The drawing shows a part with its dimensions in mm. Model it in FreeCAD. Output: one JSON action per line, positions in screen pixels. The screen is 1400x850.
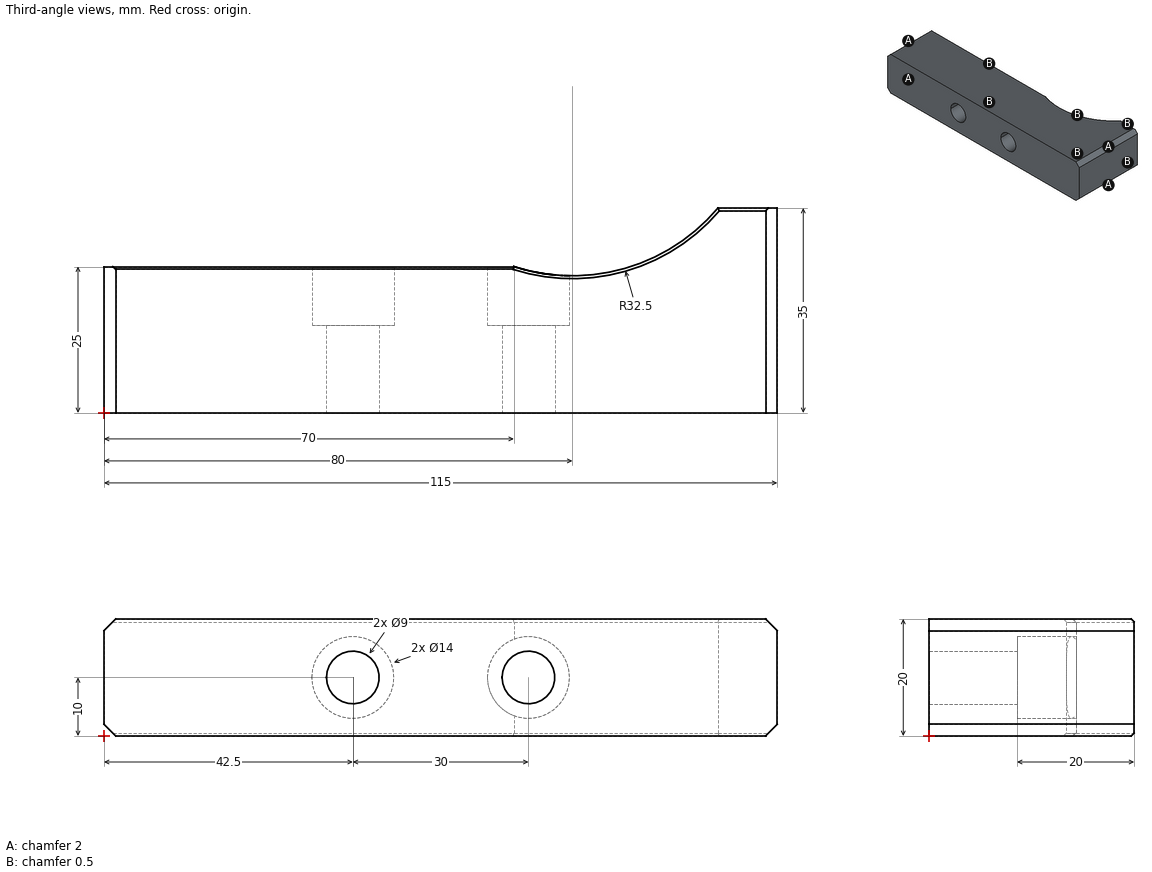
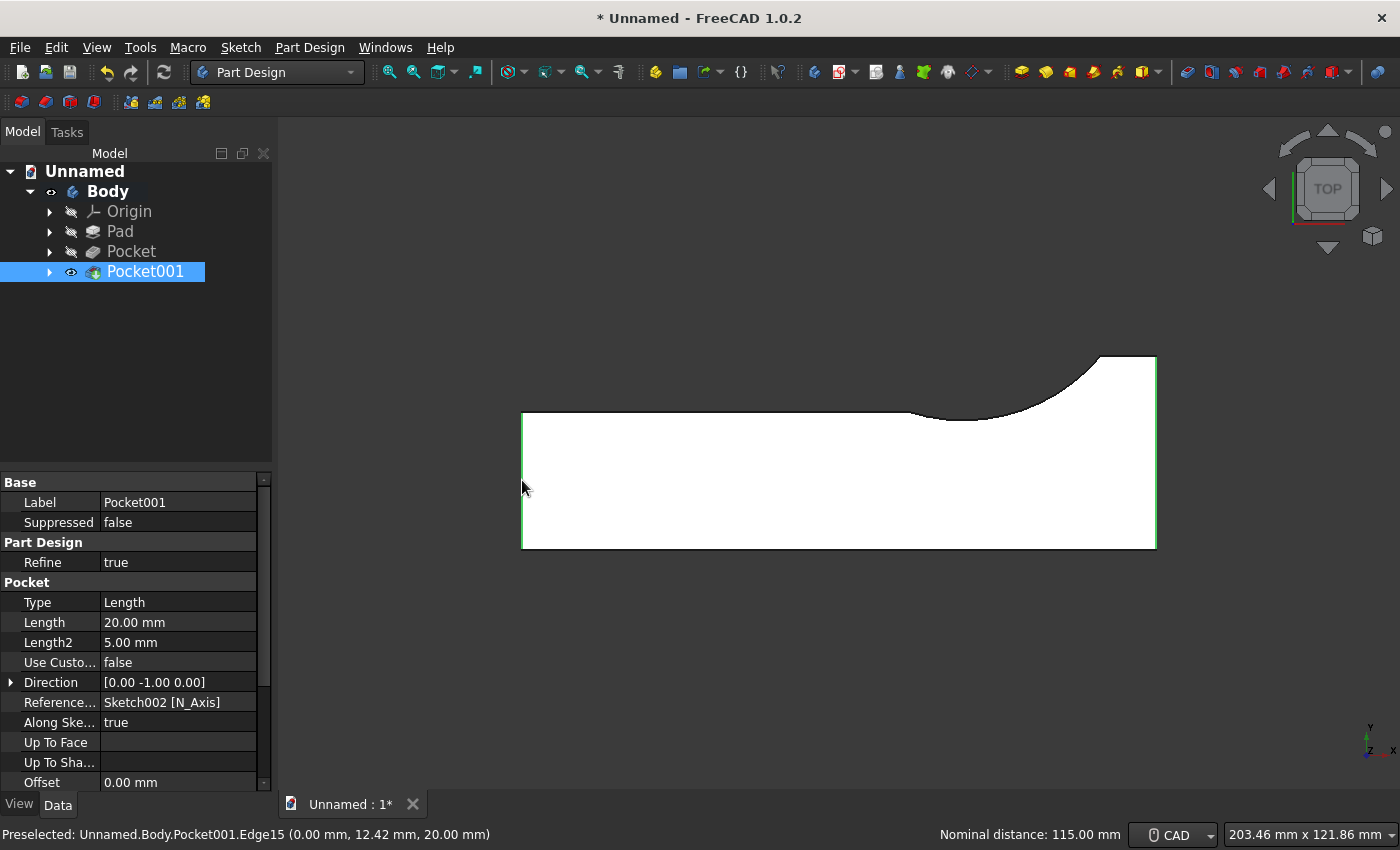
{"action": "key", "text": "1"}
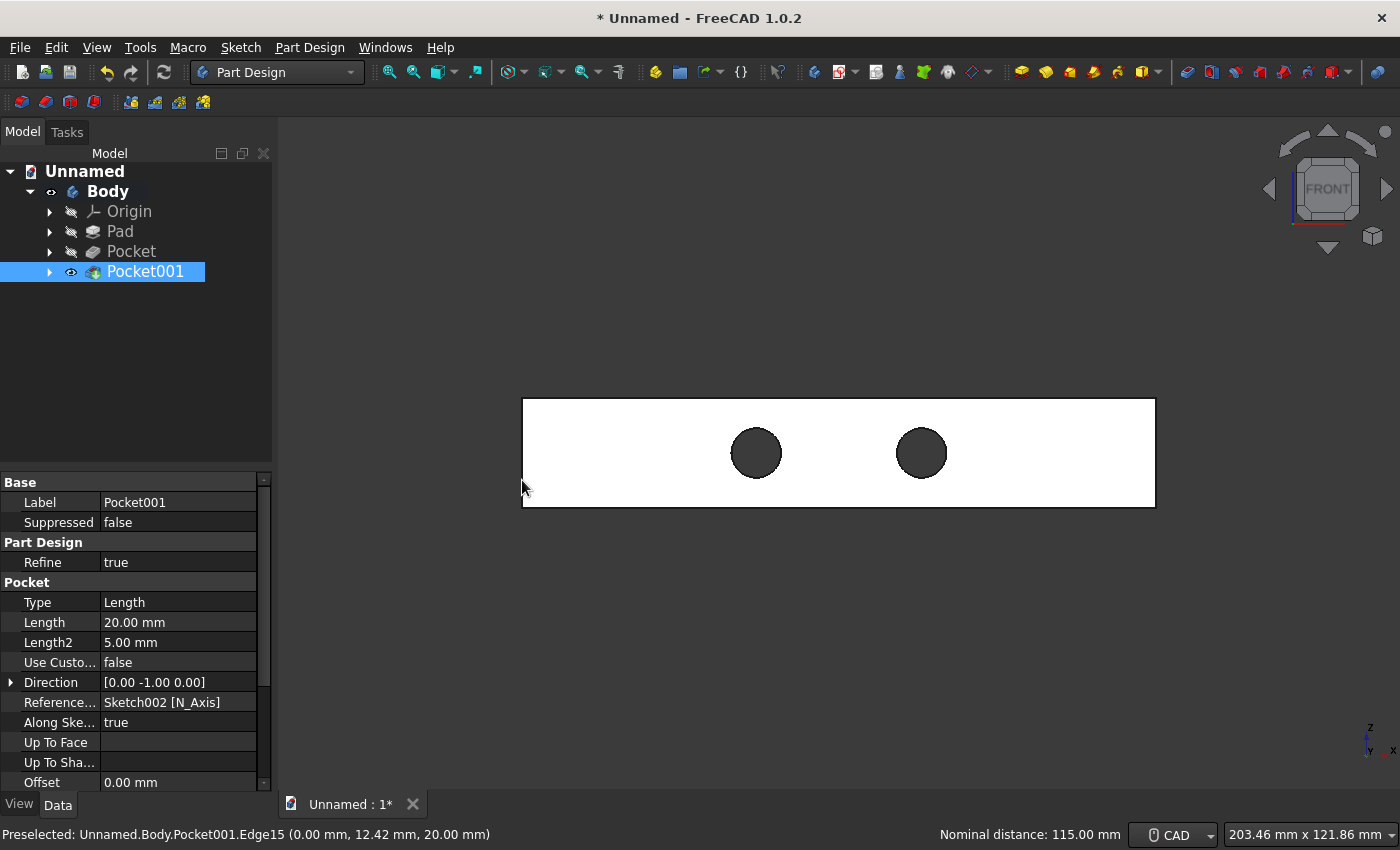
{"action": "key", "text": "3"}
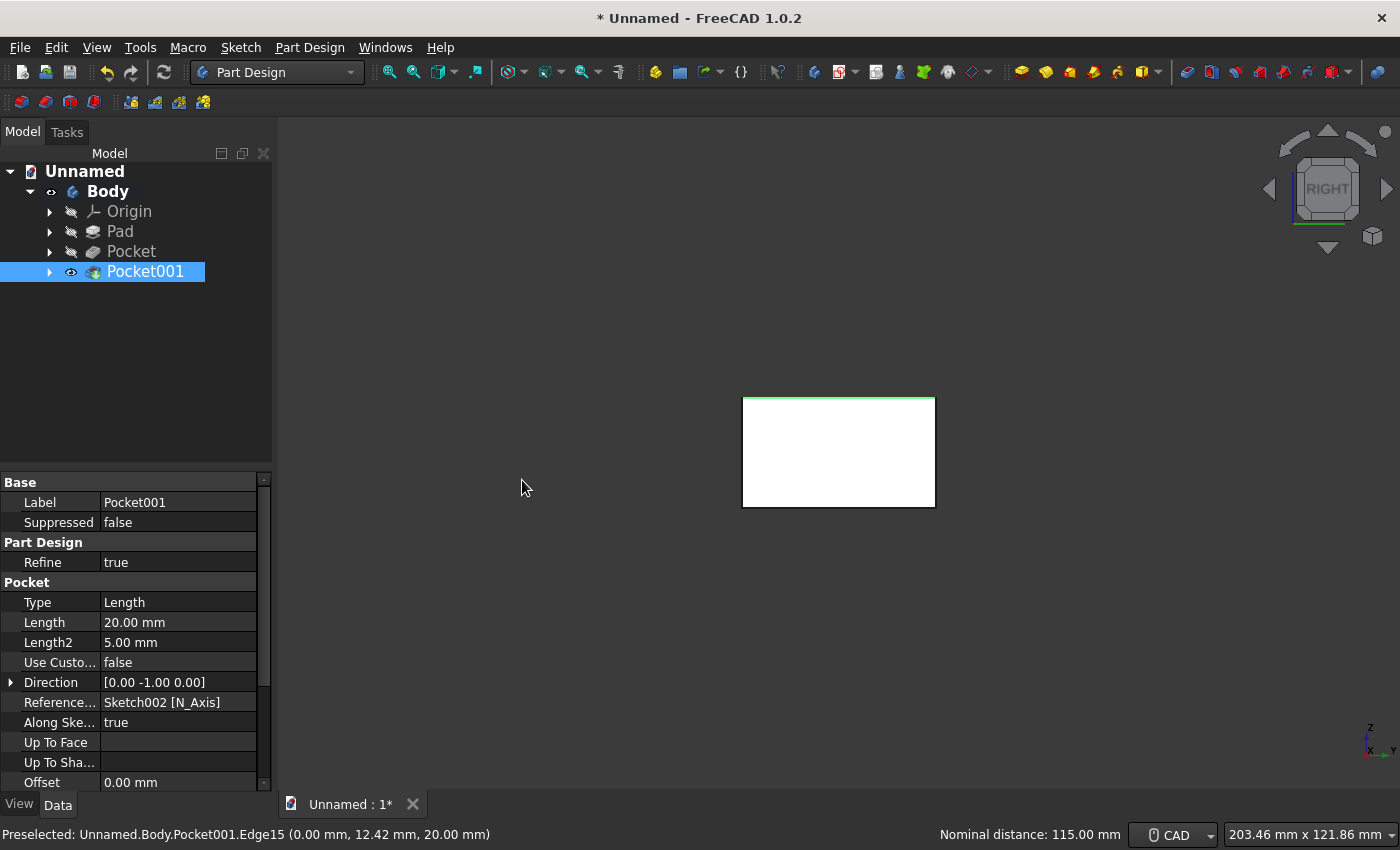
{"action": "left_click", "coordinate": [390, 72]}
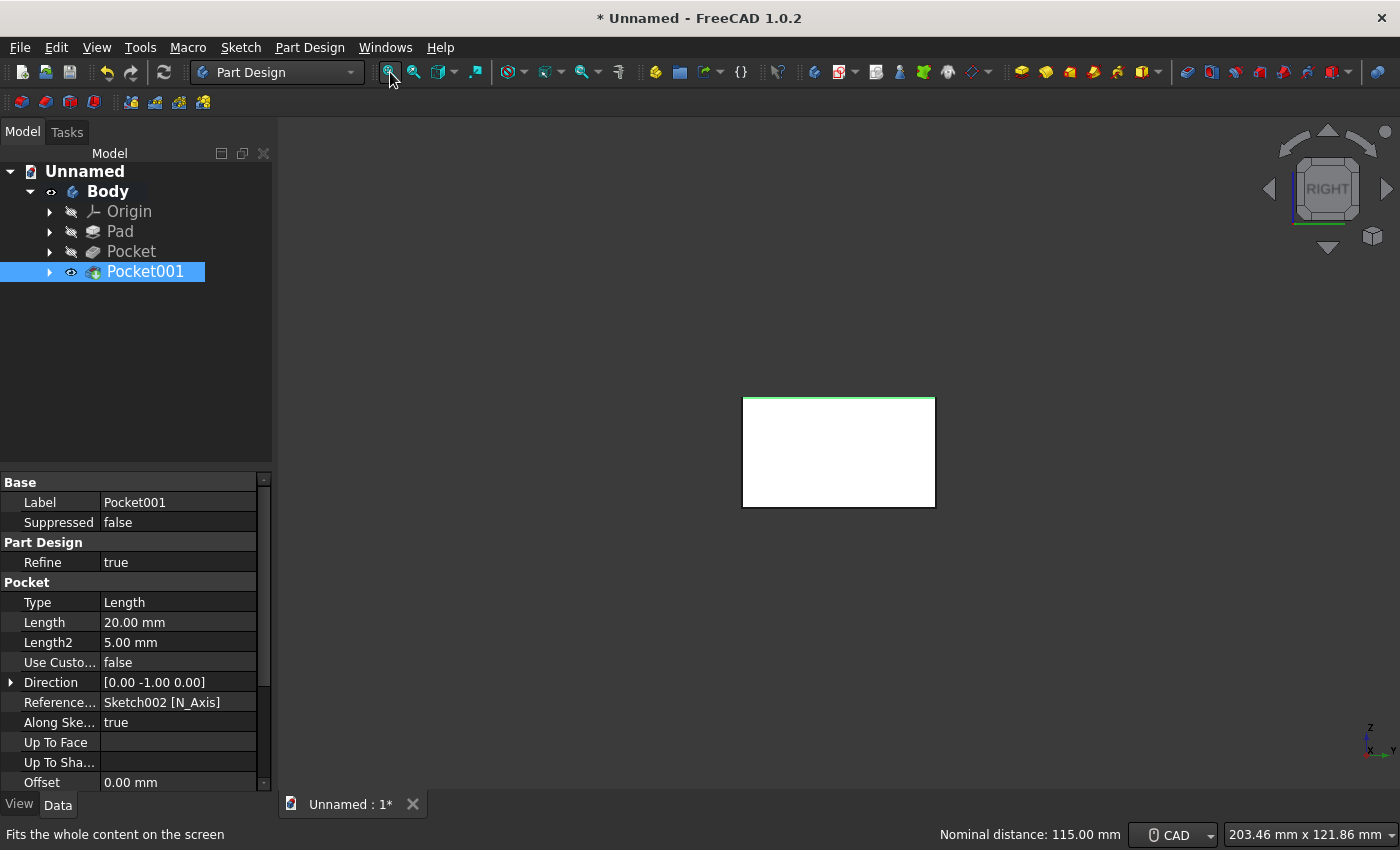
{"action": "left_click", "coordinate": [839, 507], "text": "ctrl"}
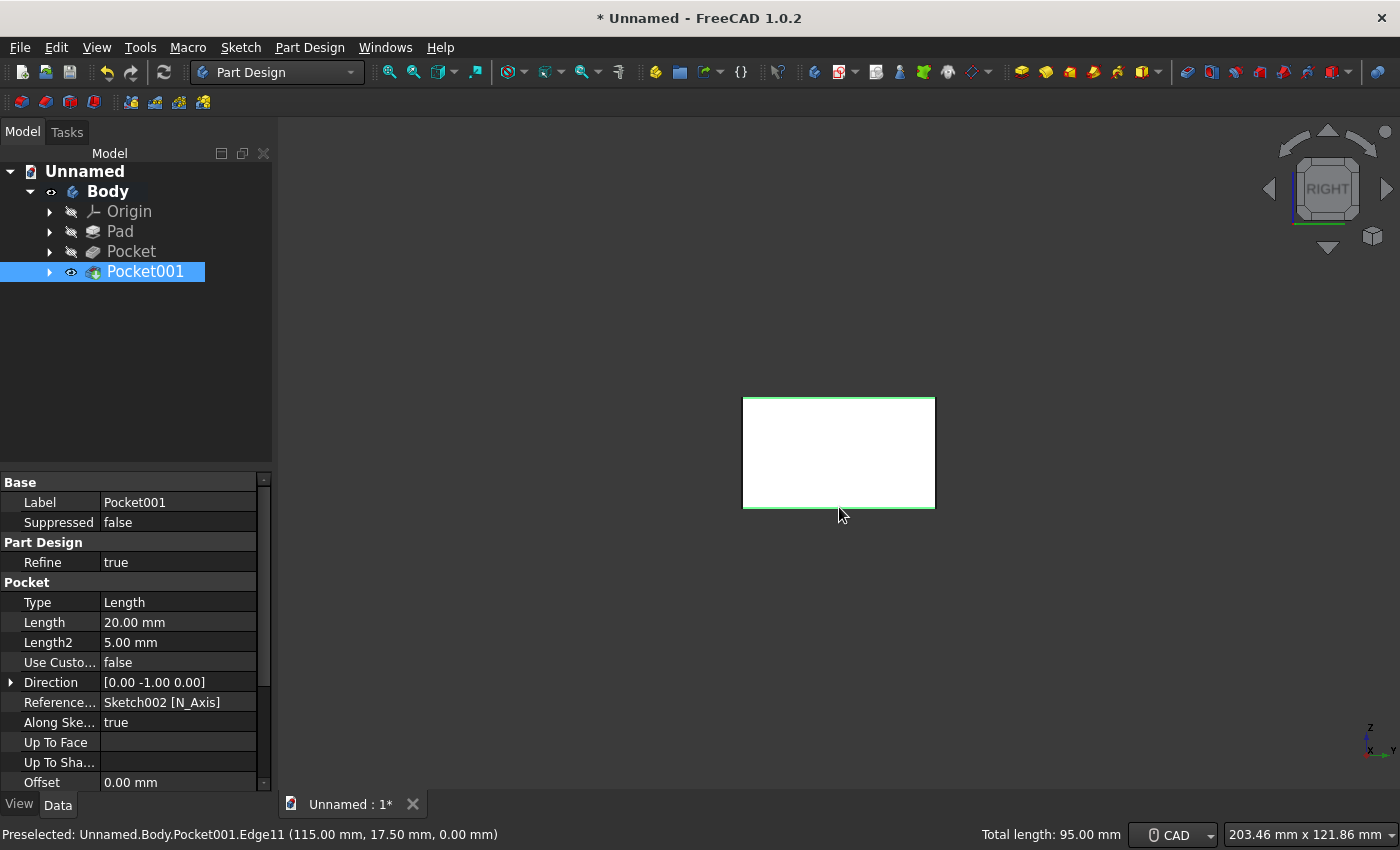
{"action": "key", "text": "5"}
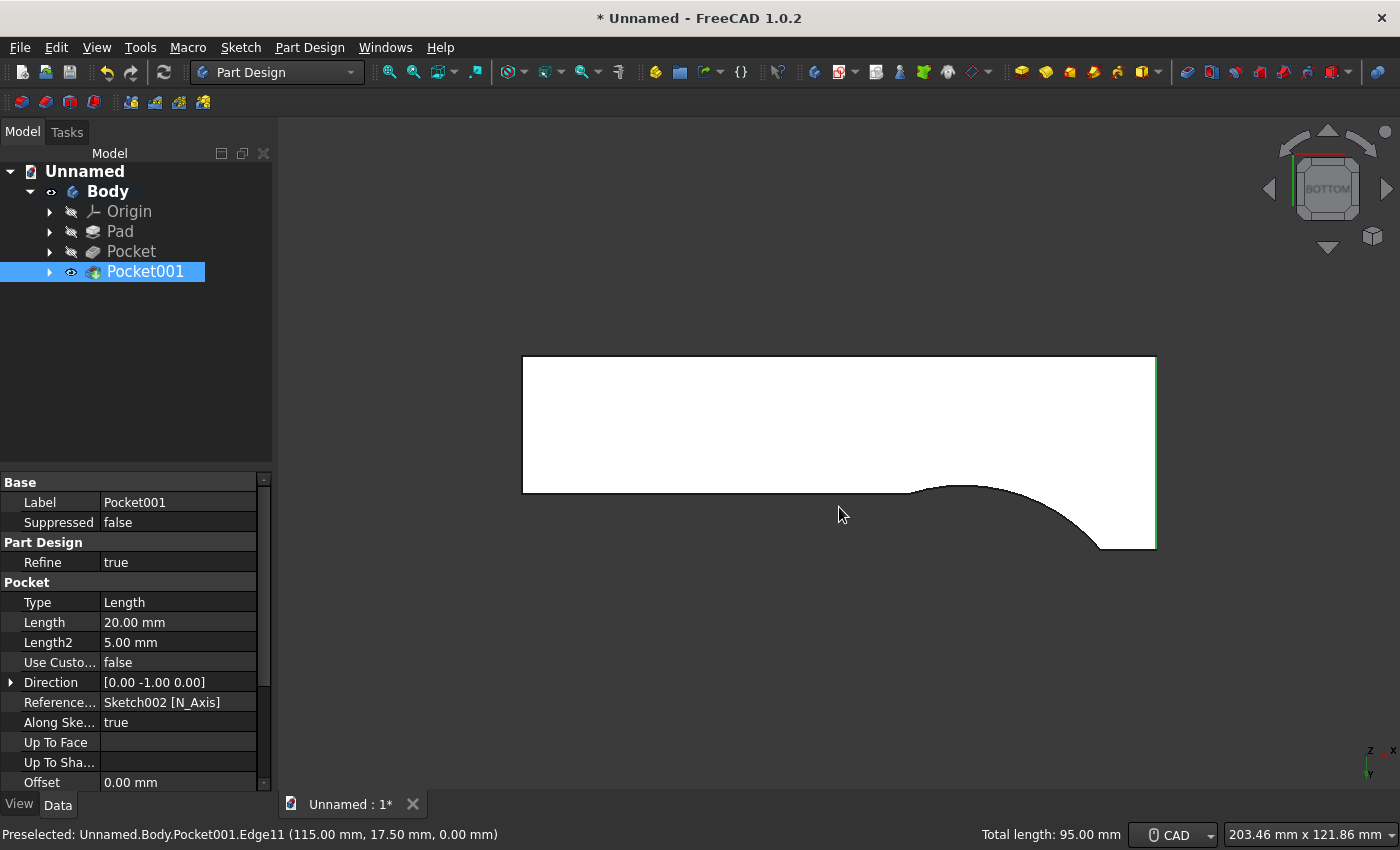
{"action": "left_click", "coordinate": [522, 424], "text": "ctrl"}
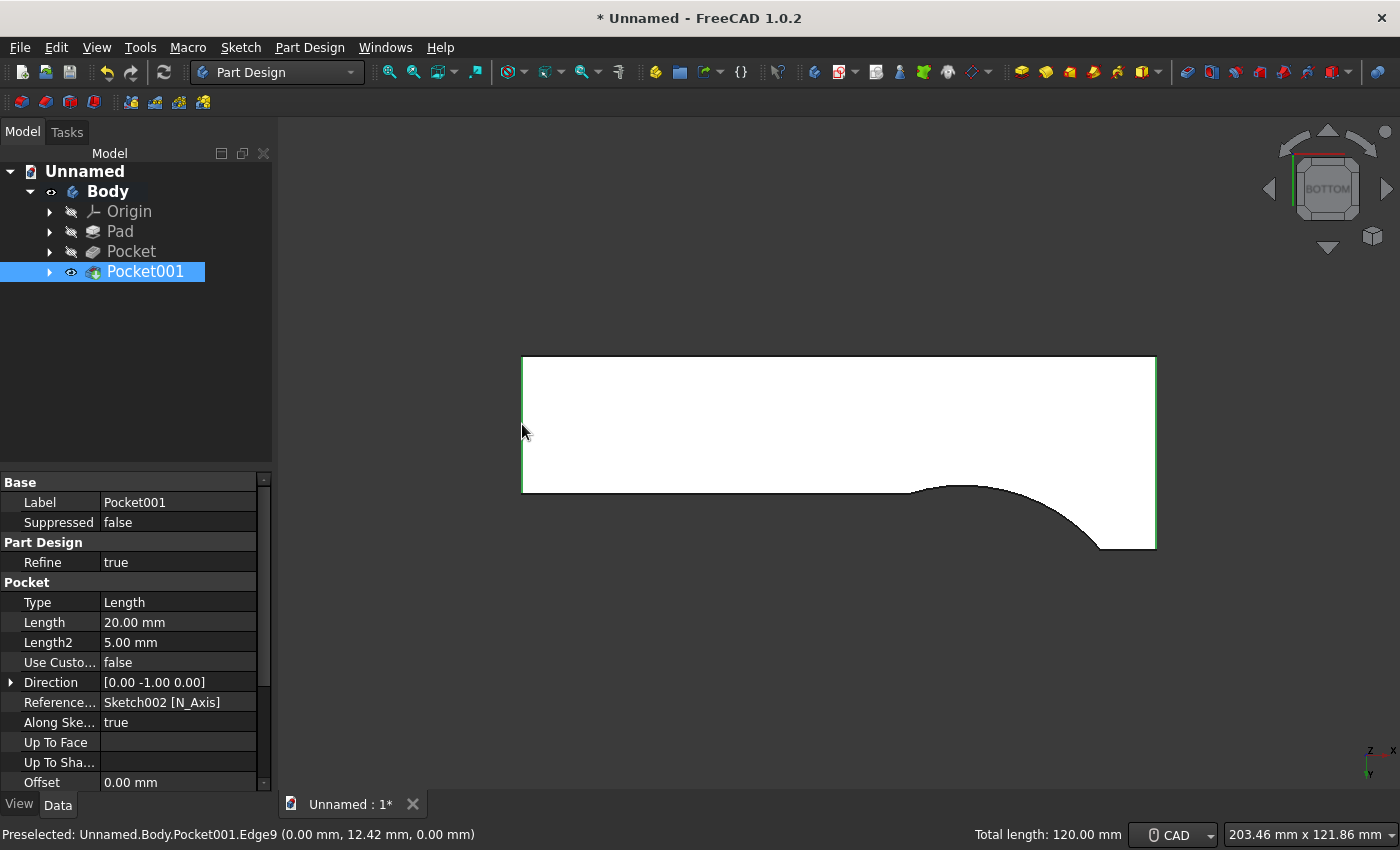
{"action": "left_click", "coordinate": [46, 102]}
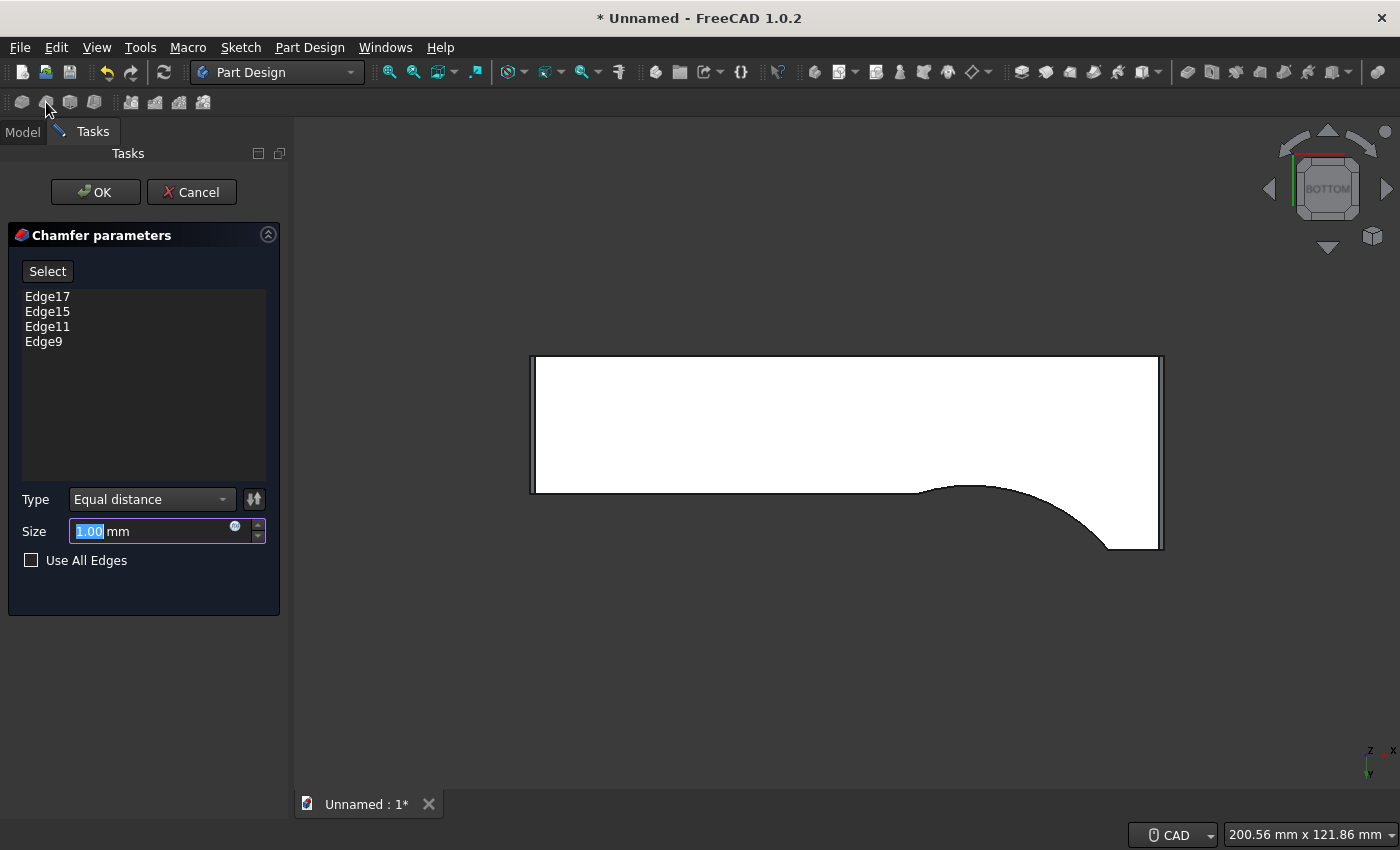
{"action": "type", "text": "2"}
{"action": "key", "text": "Tab"}